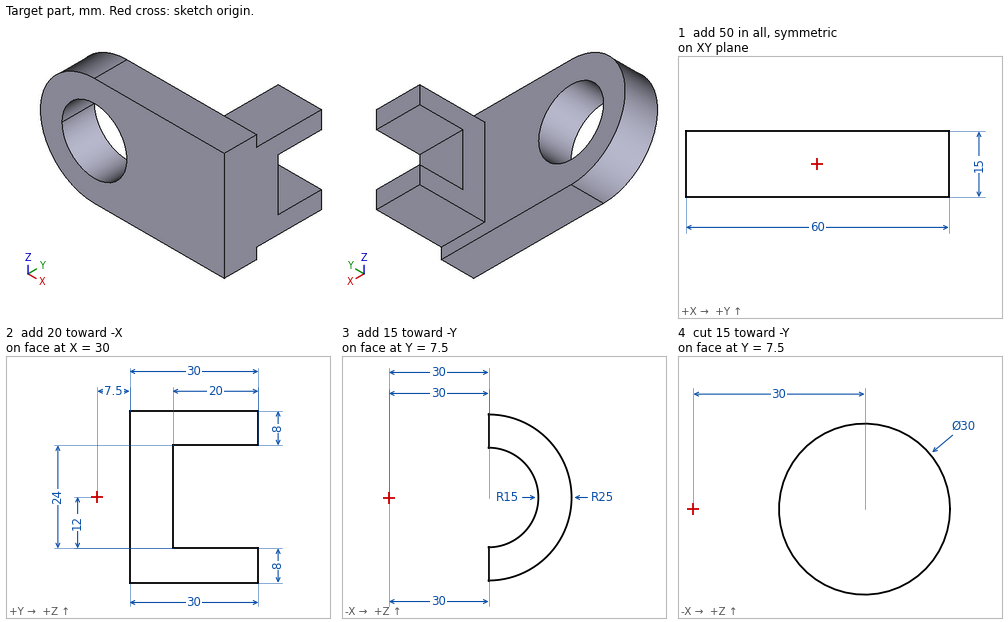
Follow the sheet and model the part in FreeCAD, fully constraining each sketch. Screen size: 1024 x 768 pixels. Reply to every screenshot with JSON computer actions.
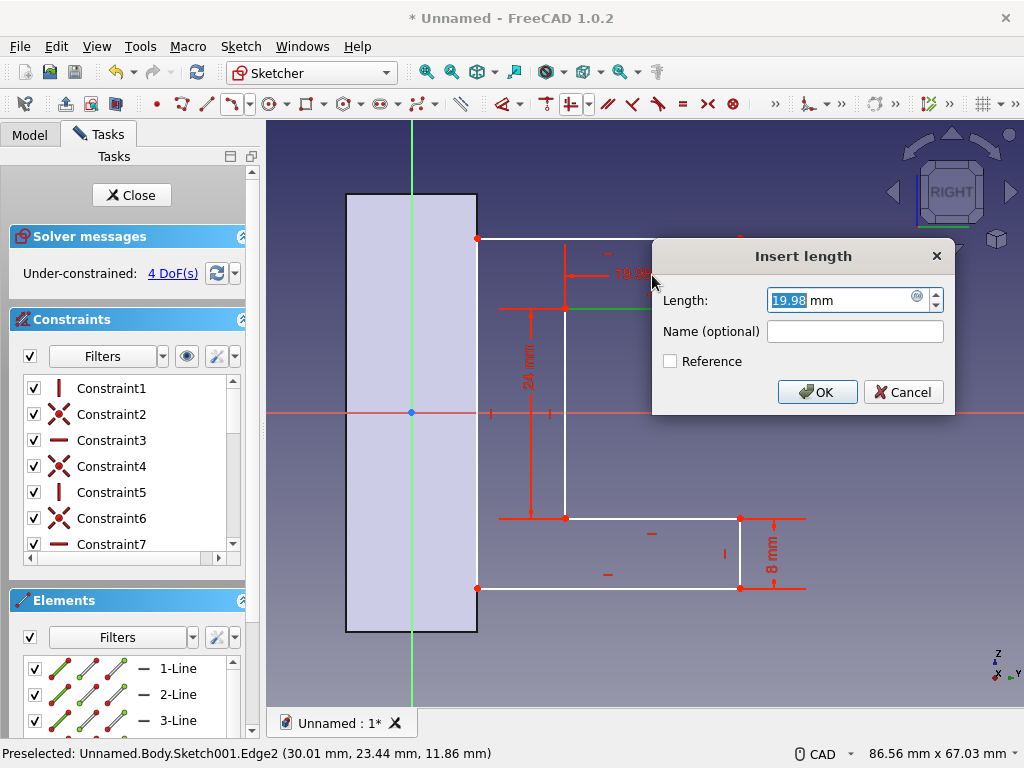
{"action": "type", "text": "20"}
{"action": "key", "text": "Return"}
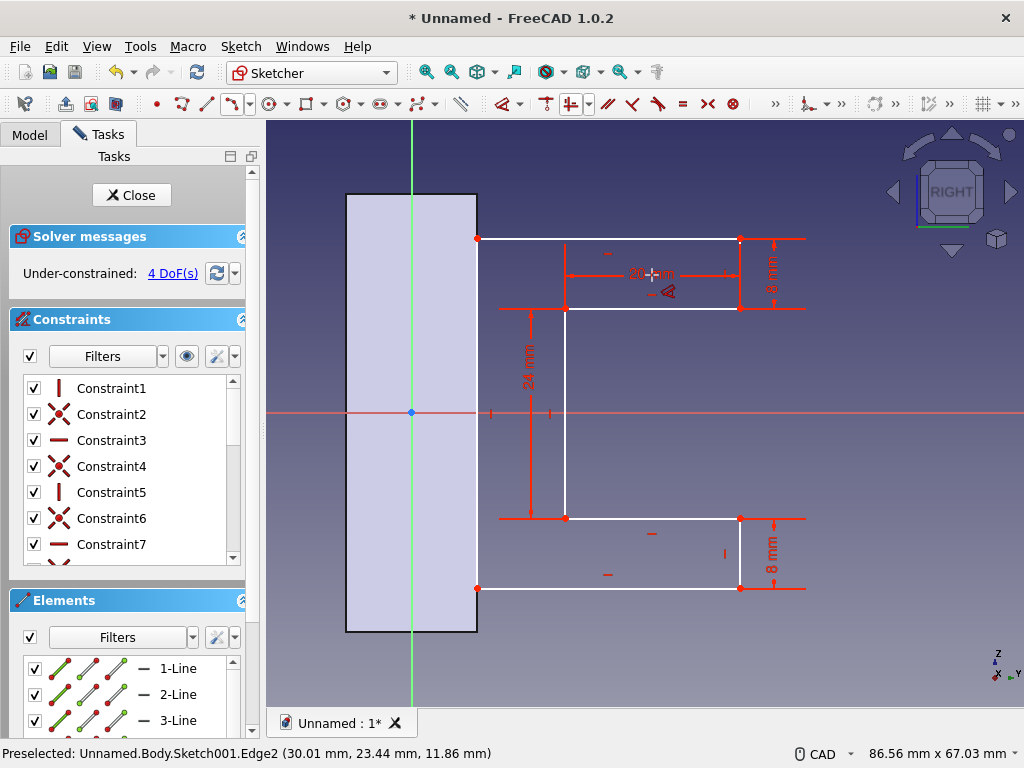
{"action": "left_click", "coordinate": [661, 239]}
{"action": "left_click", "coordinate": [609, 205]}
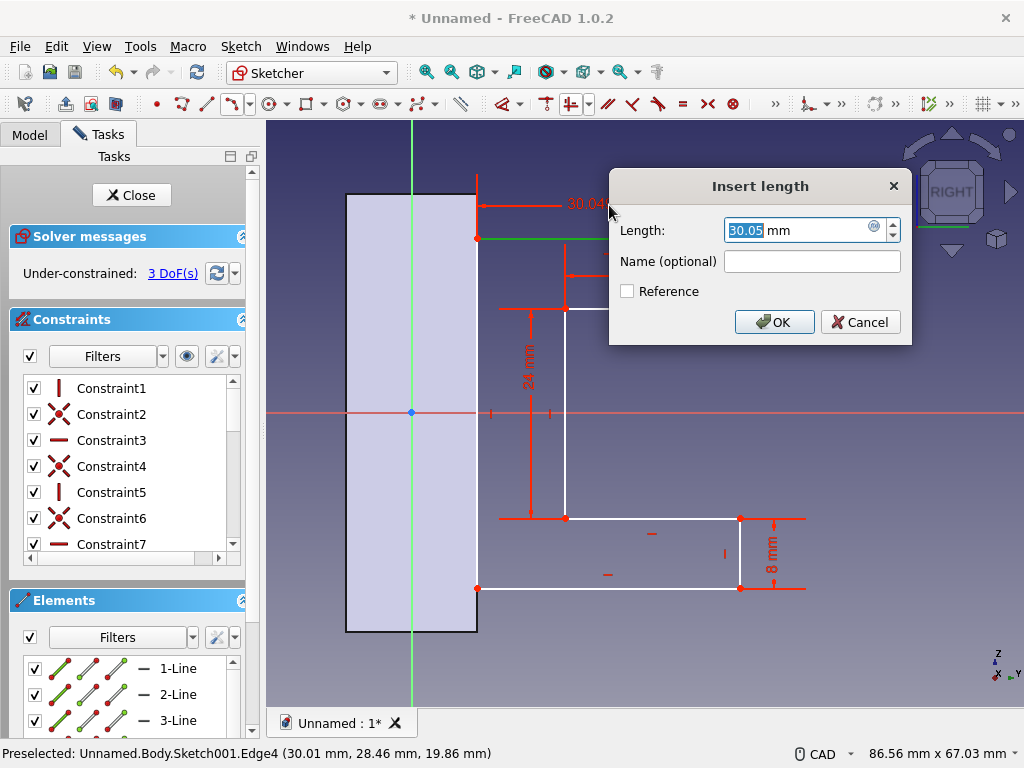
{"action": "type", "text": "30"}
{"action": "key", "text": "Return"}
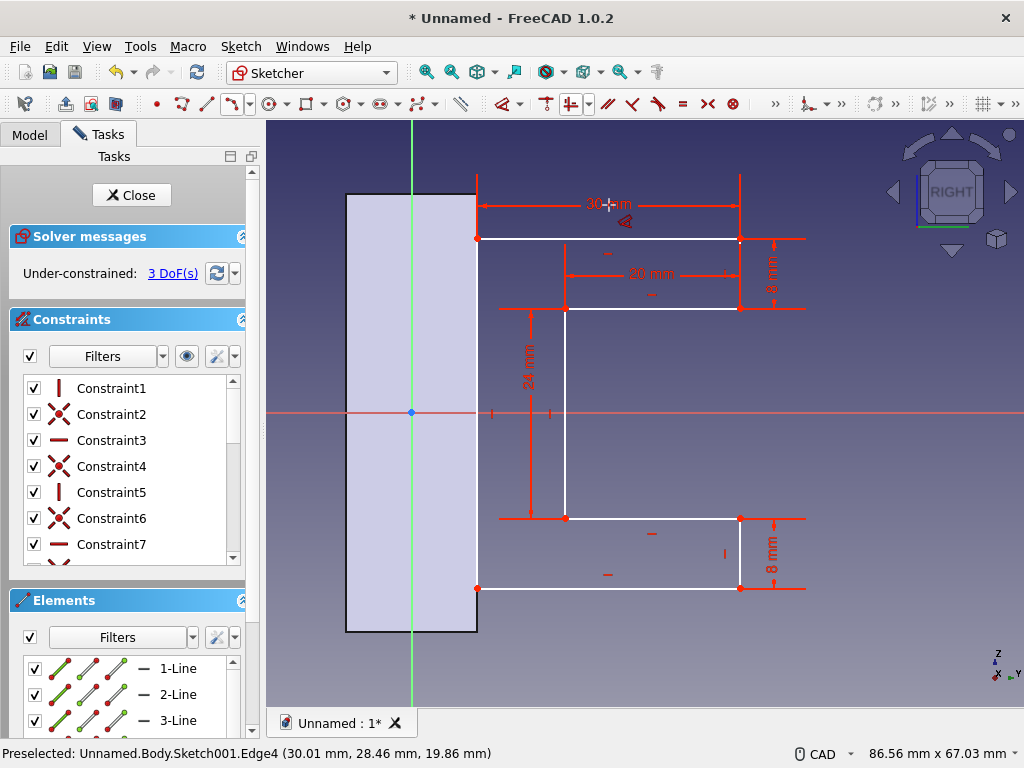
{"action": "left_click", "coordinate": [556, 589]}
{"action": "left_click", "coordinate": [609, 623]}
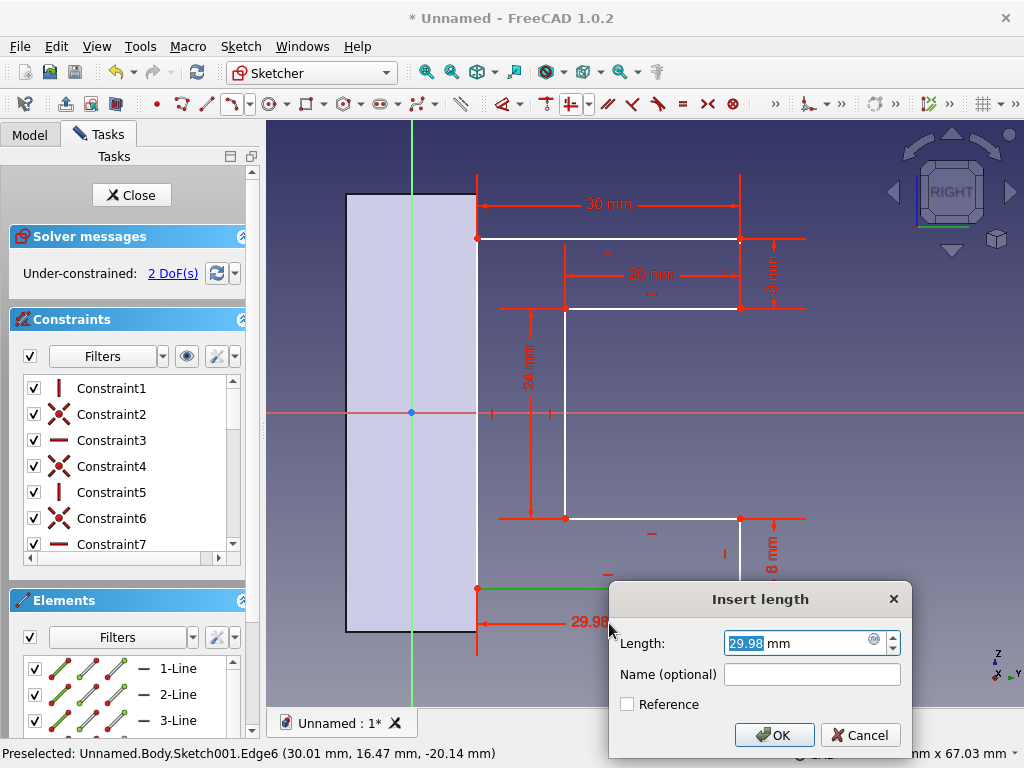
{"action": "type", "text": "30"}
{"action": "key", "text": "Return"}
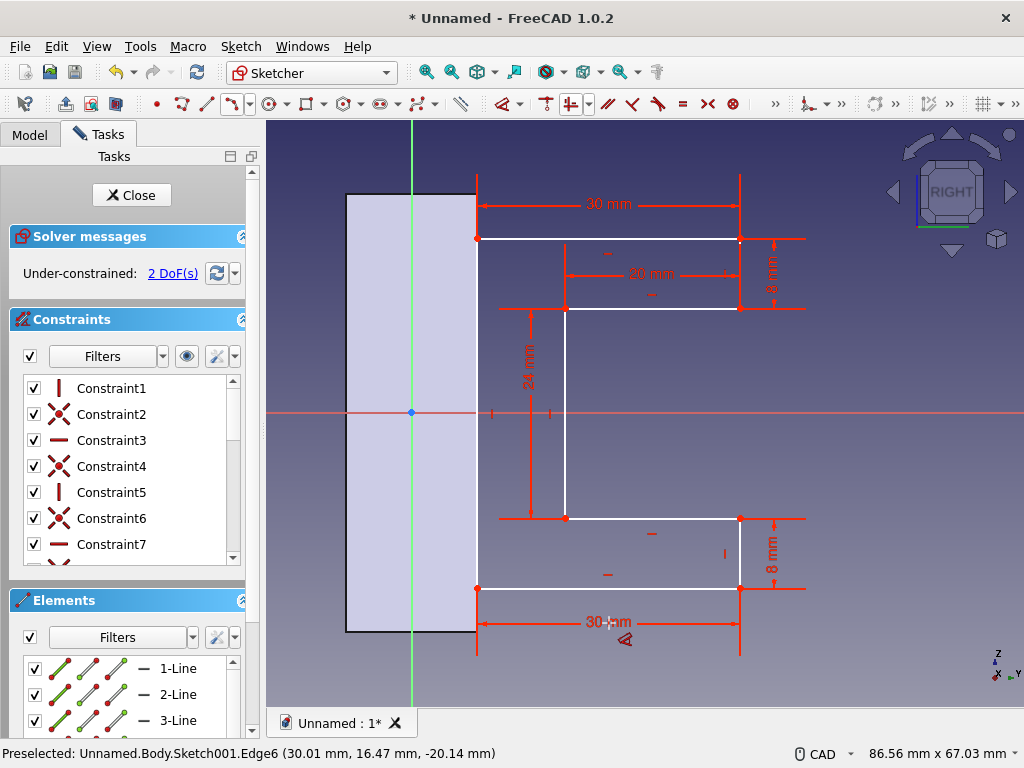
{"action": "left_click", "coordinate": [565, 519]}
{"action": "left_click", "coordinate": [378, 466]}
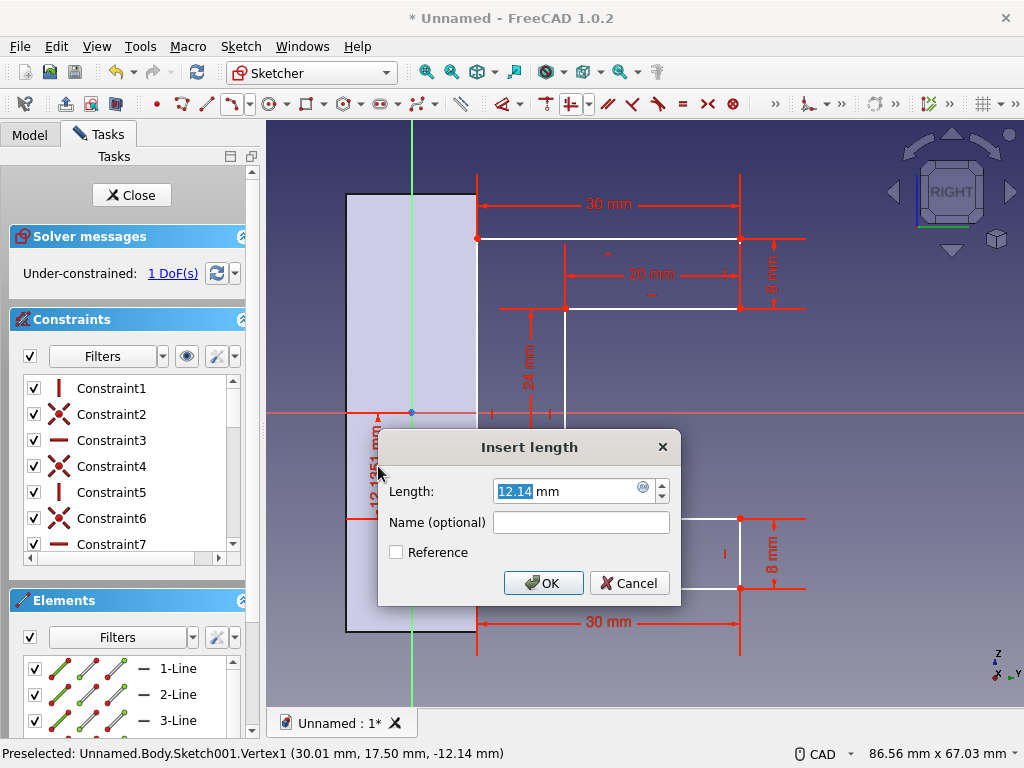
{"action": "type", "text": "12"}
{"action": "key", "text": "Return"}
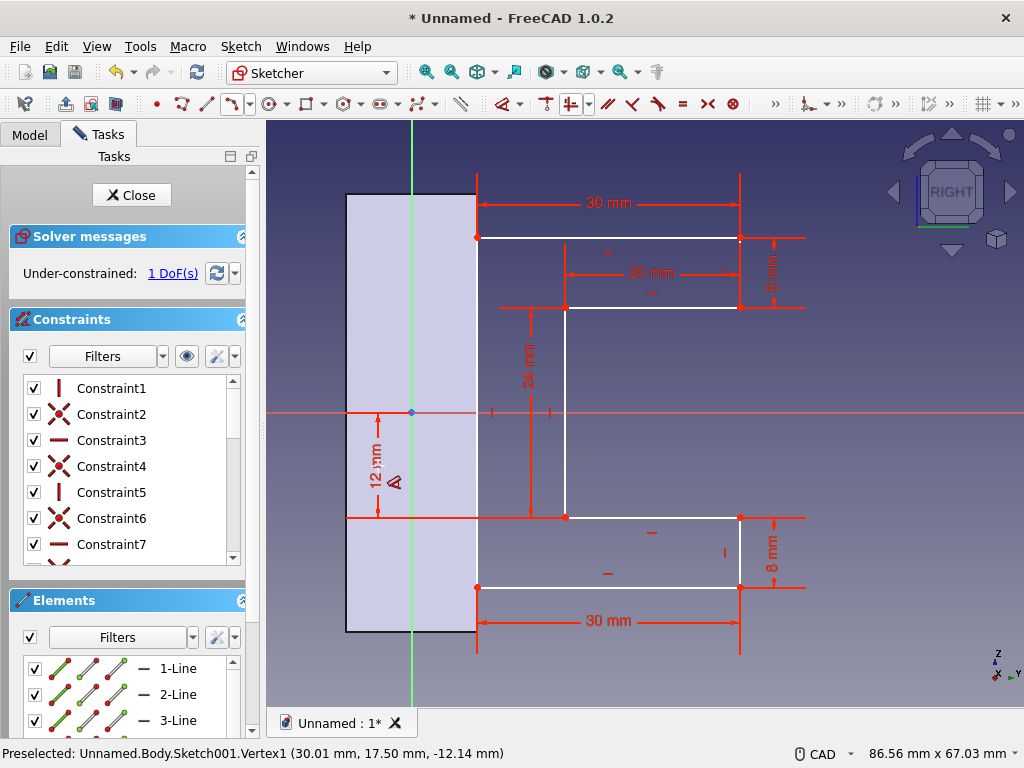
{"action": "left_click", "coordinate": [477, 238]}
{"action": "left_click", "coordinate": [445, 204]}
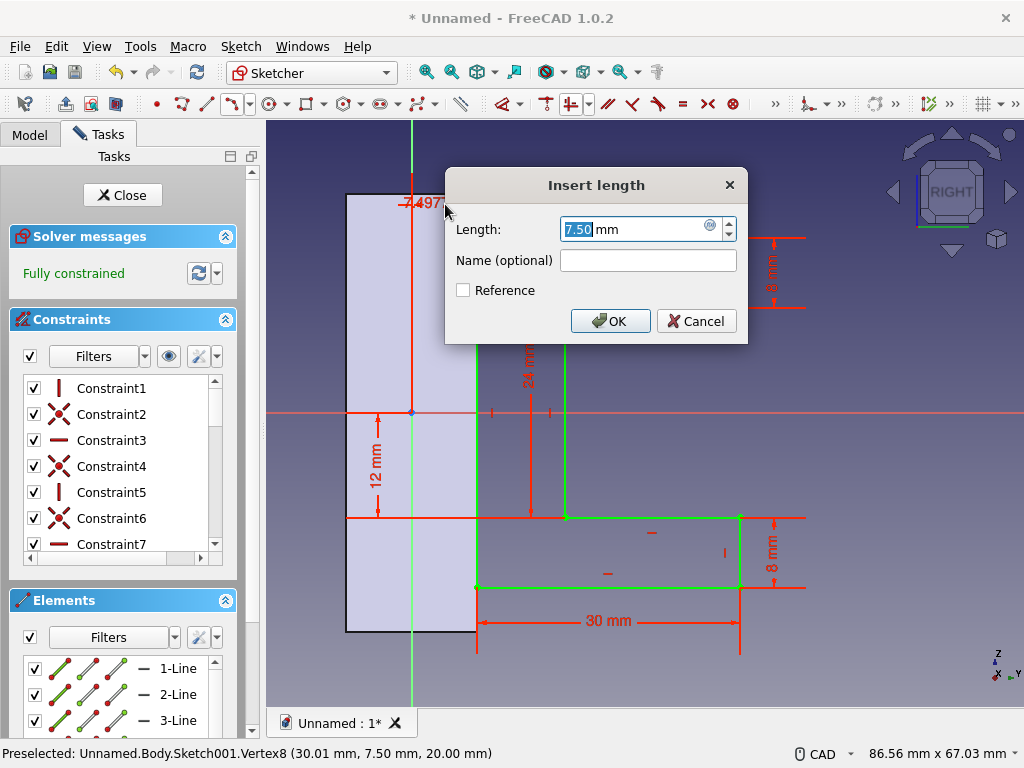
{"action": "type", "text": "7.5"}
{"action": "key", "text": "Return"}
{"action": "key", "text": "Escape"}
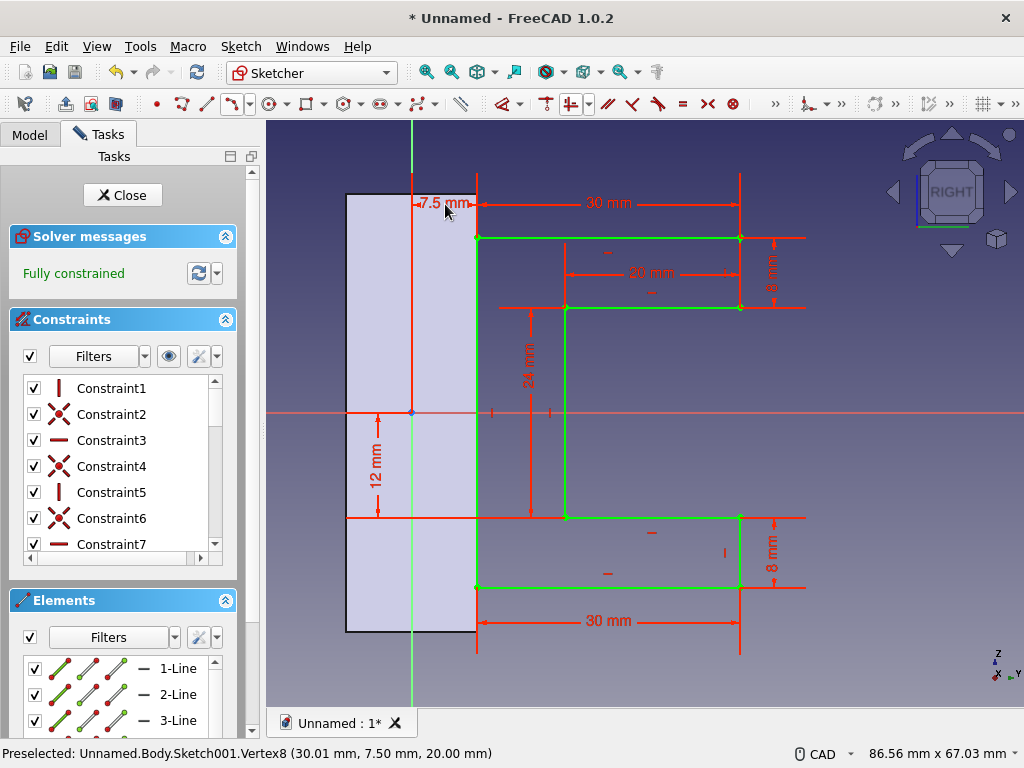
{"action": "left_click", "coordinate": [123, 195]}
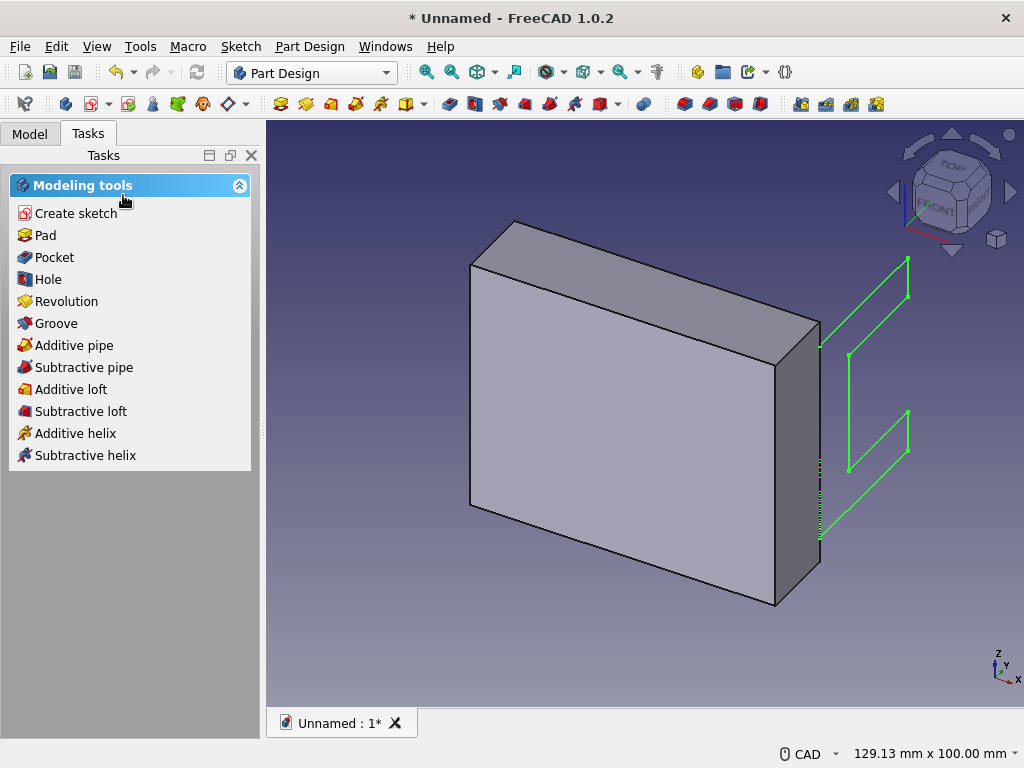
{"action": "left_click", "coordinate": [281, 104]}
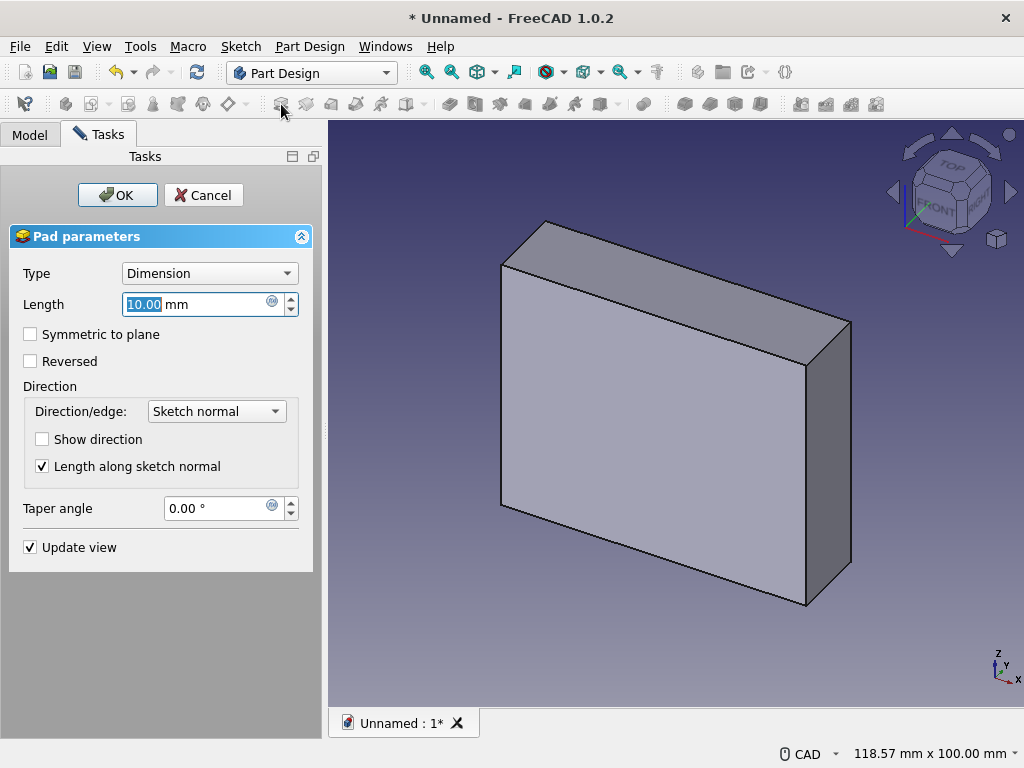
{"action": "type", "text": "20"}
{"action": "key", "text": "Tab"}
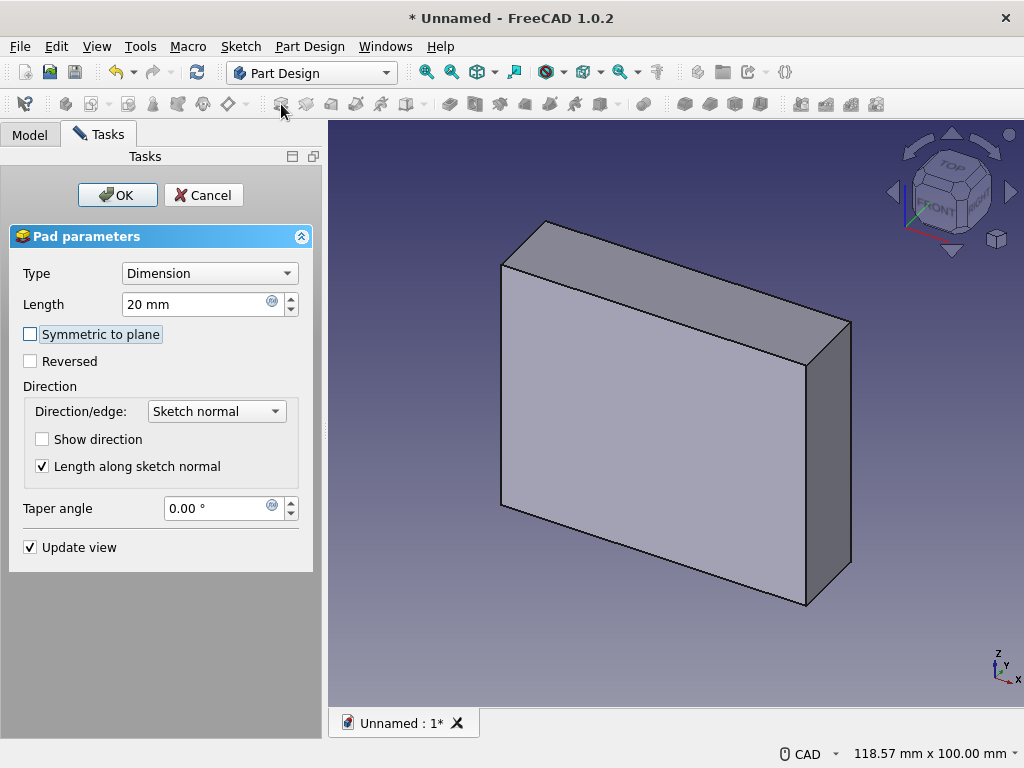
{"action": "left_click", "coordinate": [31, 361]}